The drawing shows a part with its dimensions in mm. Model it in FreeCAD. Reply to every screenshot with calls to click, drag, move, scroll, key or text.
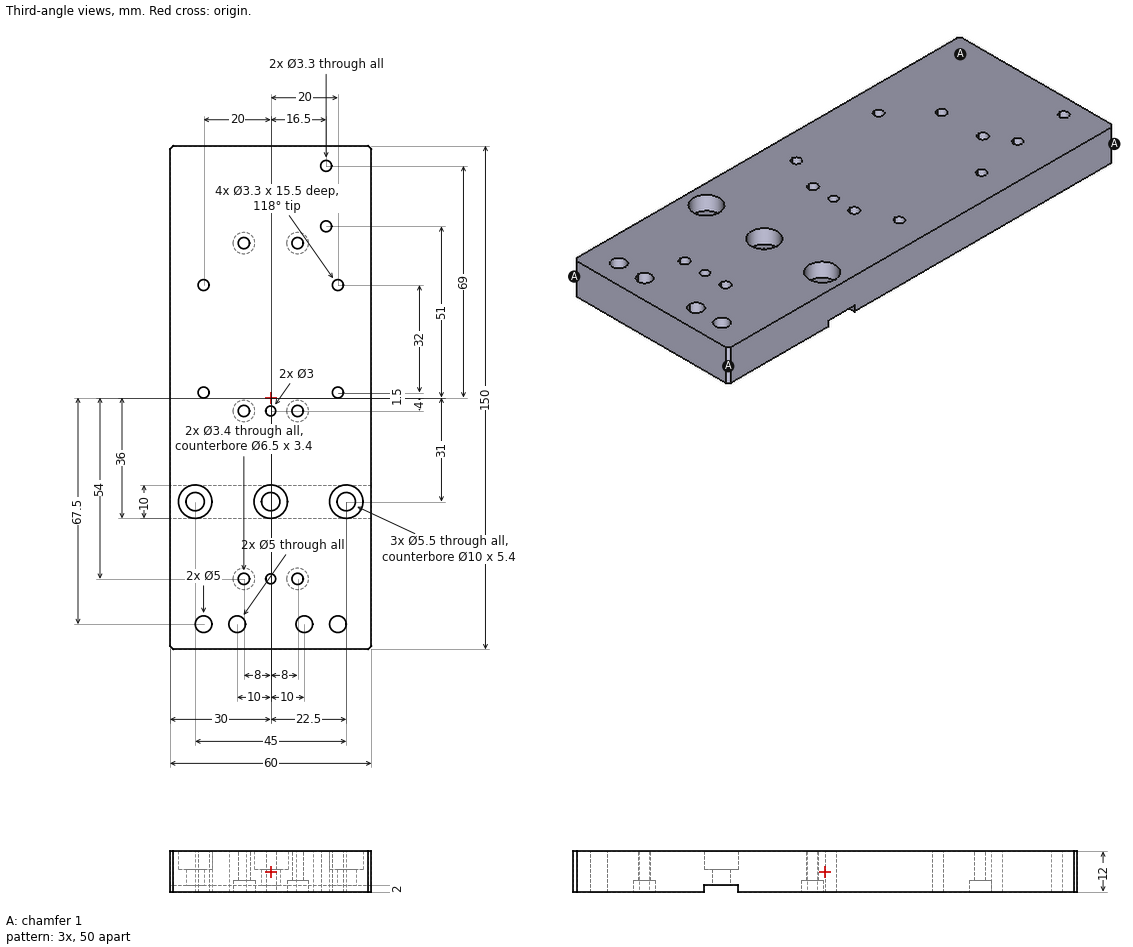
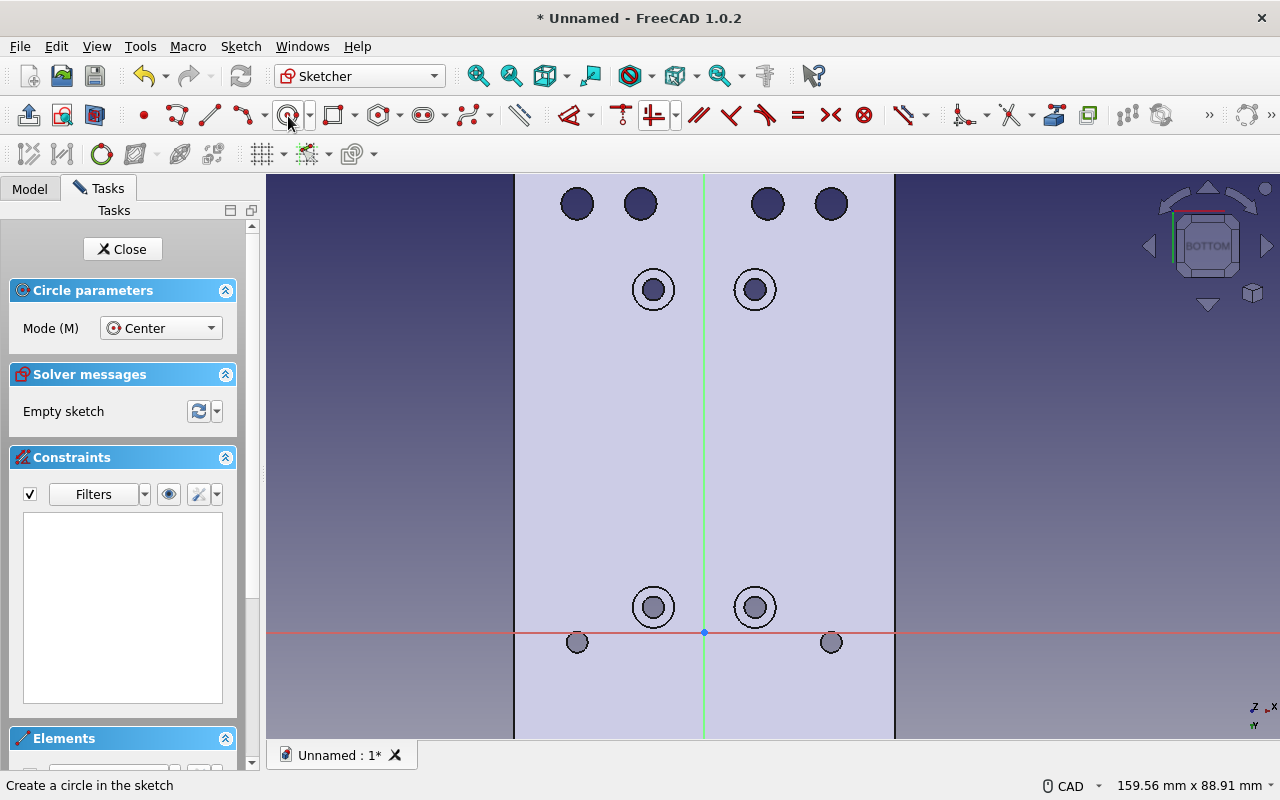
scroll(704, 607, up, 5)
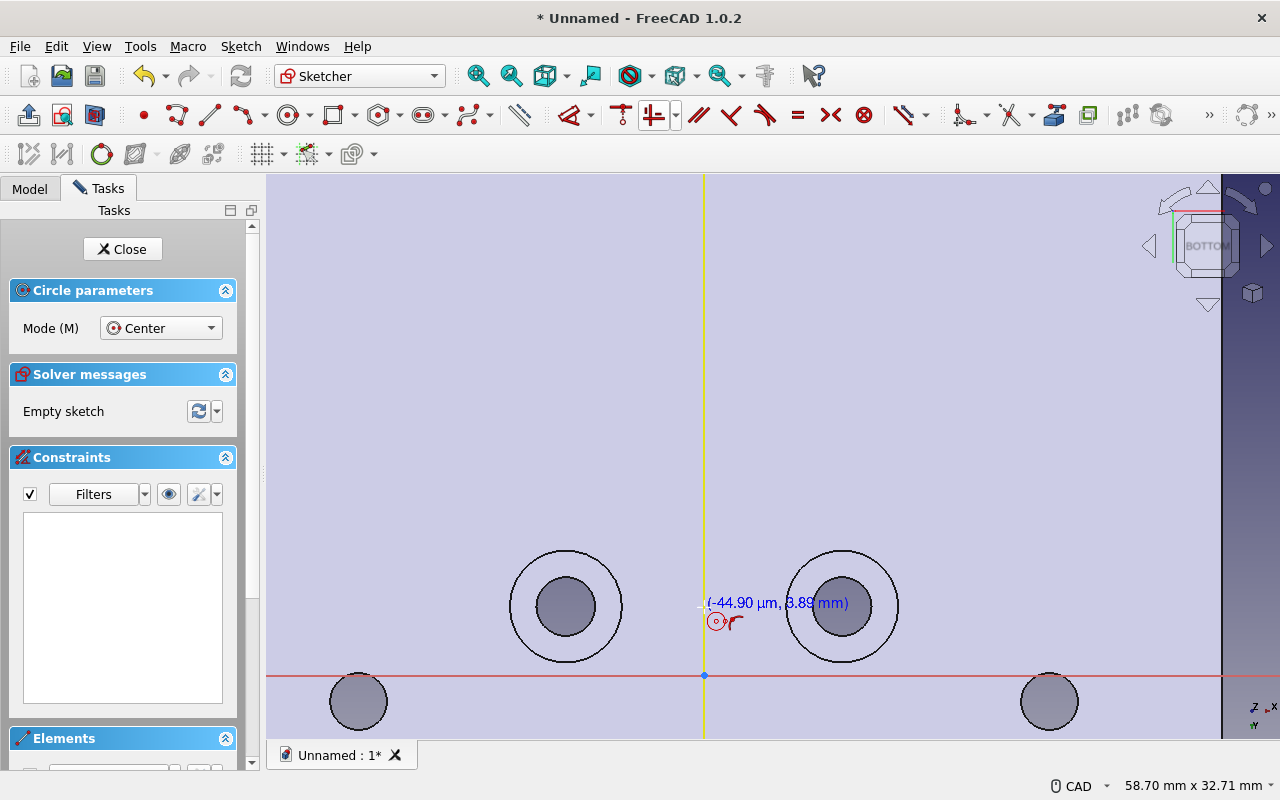
click(704, 607)
click(722, 588)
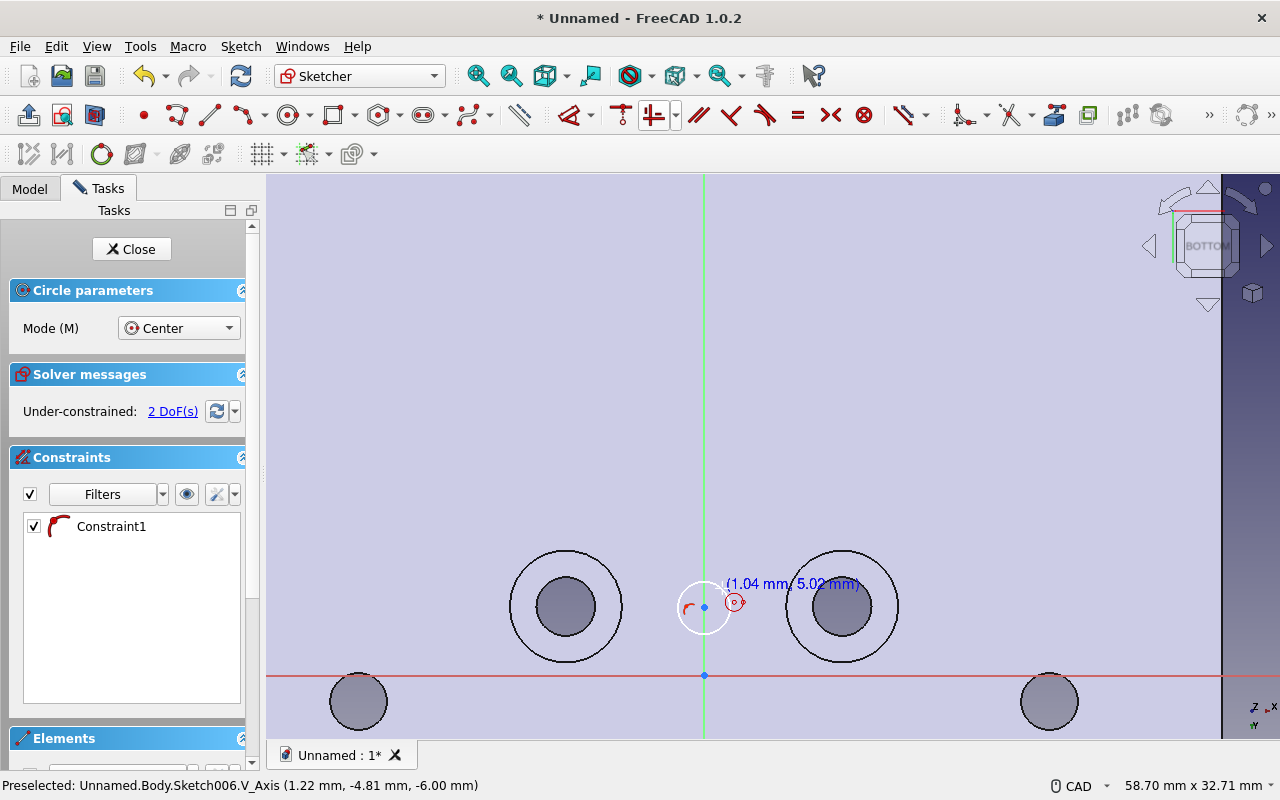
scroll(705, 608, down, 5)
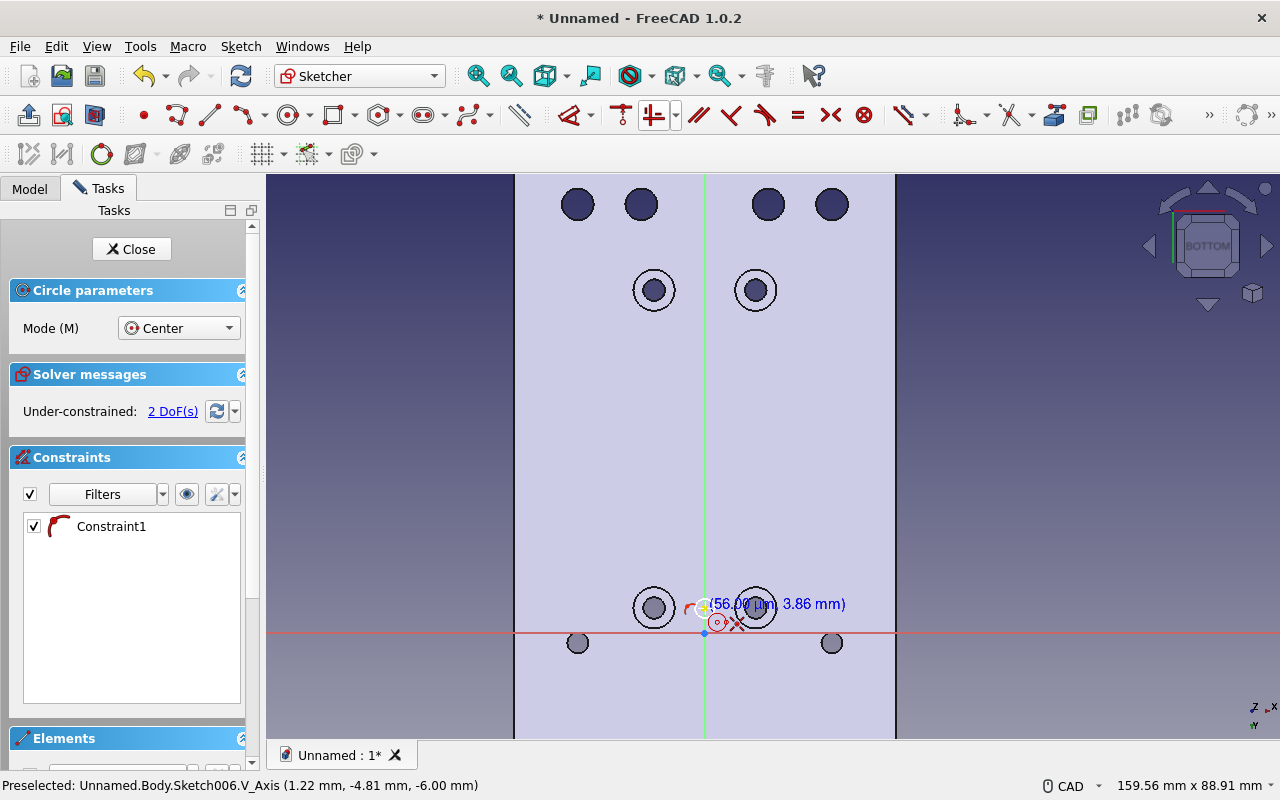
scroll(705, 290, up, 5)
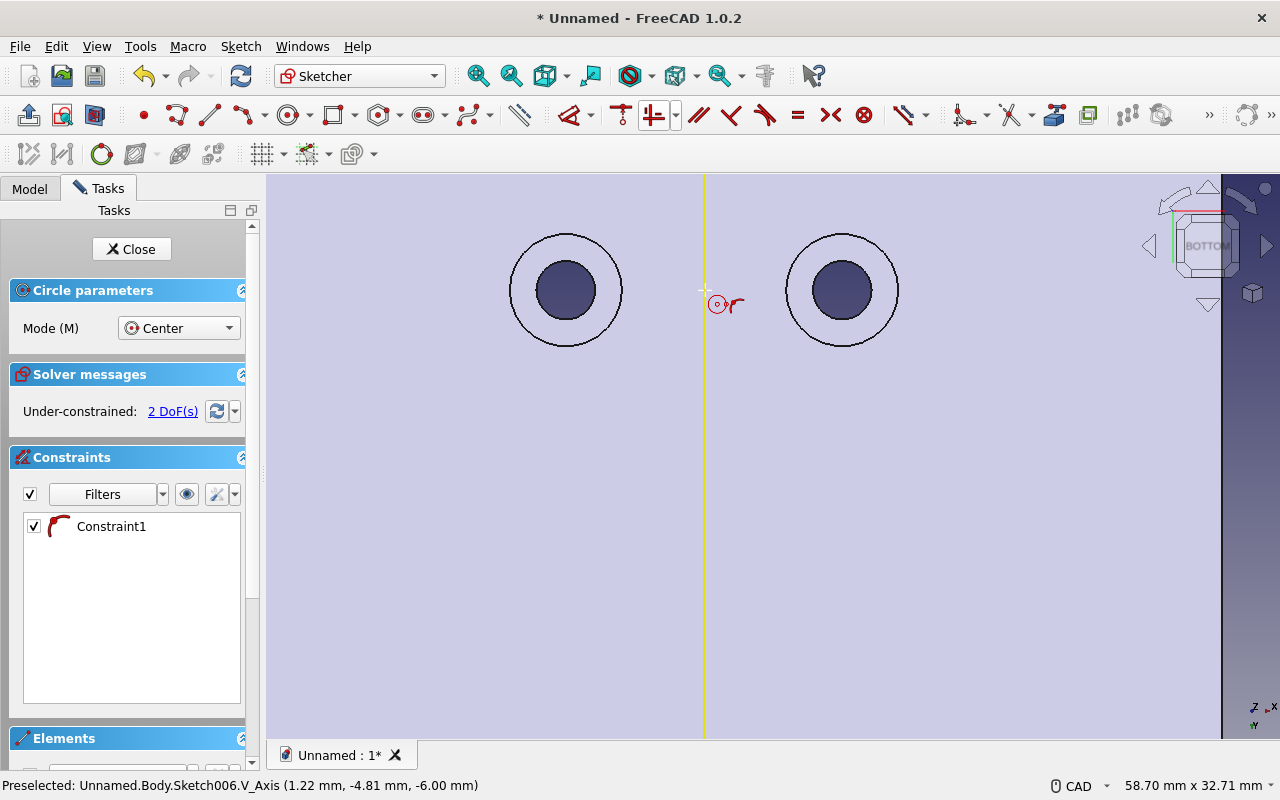
click(704, 290)
click(722, 272)
key(Escape)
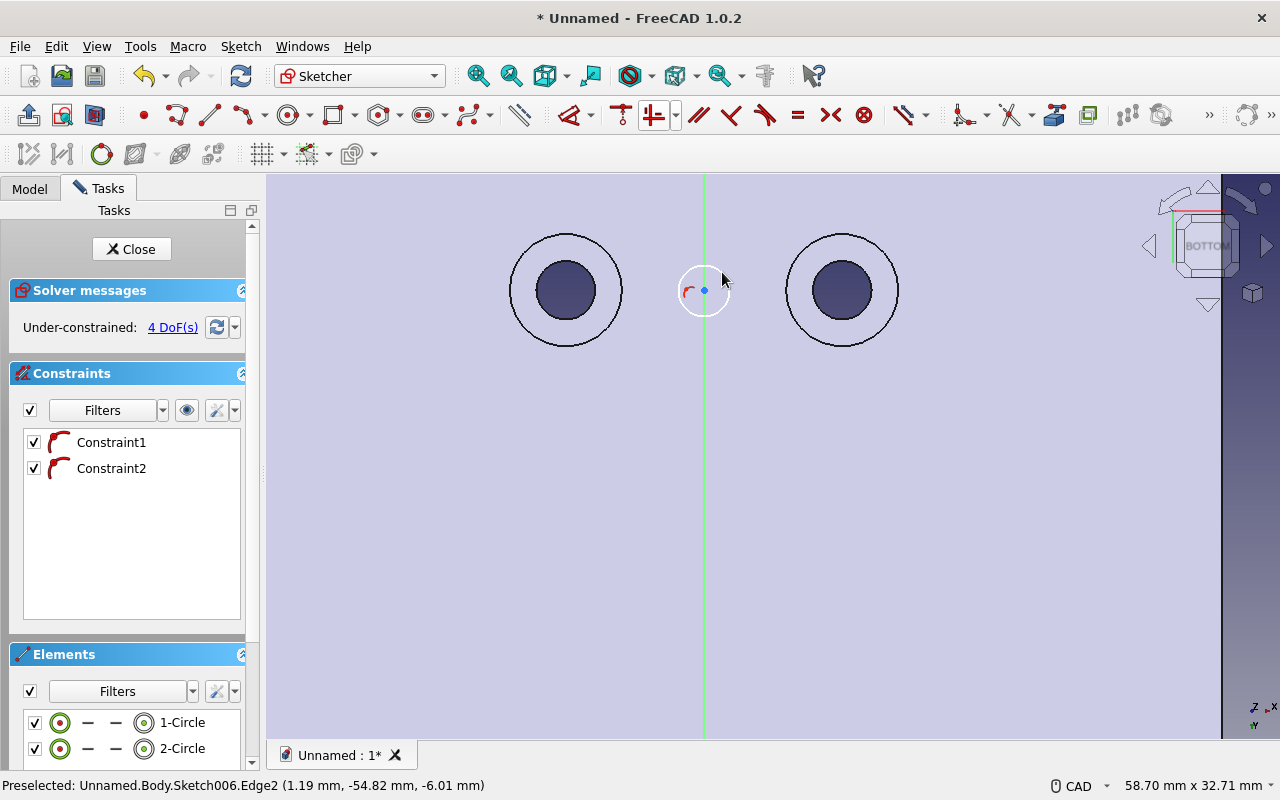
scroll(705, 289, down, 5)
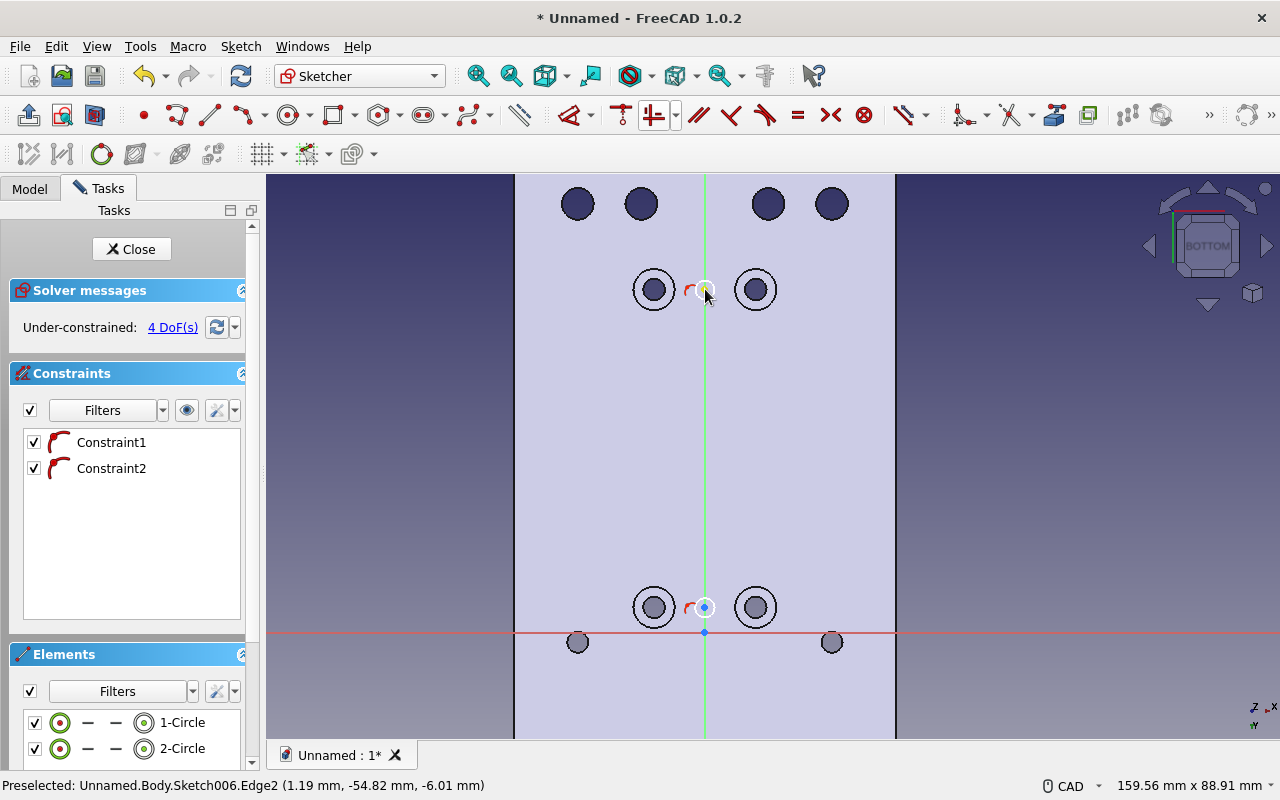
scroll(712, 601, up, 4)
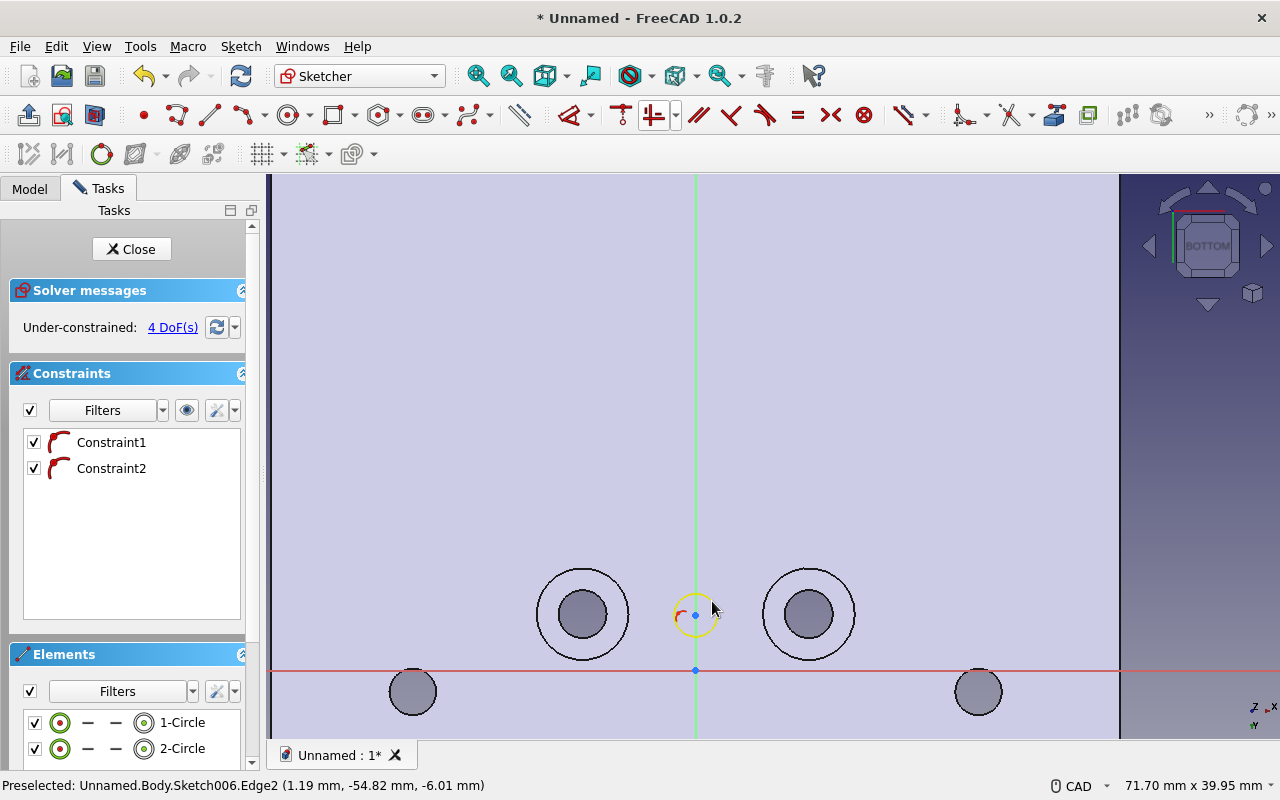
click(711, 600)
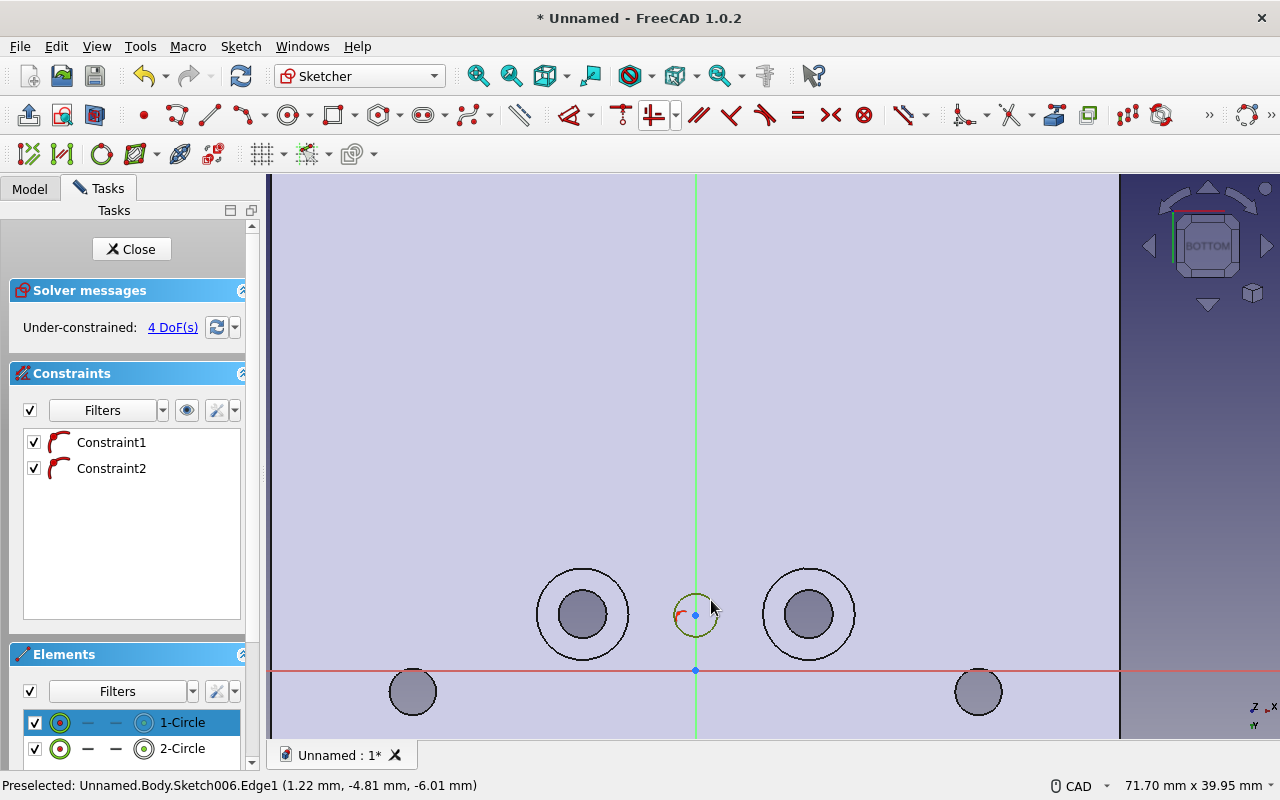
scroll(712, 602, down, 4)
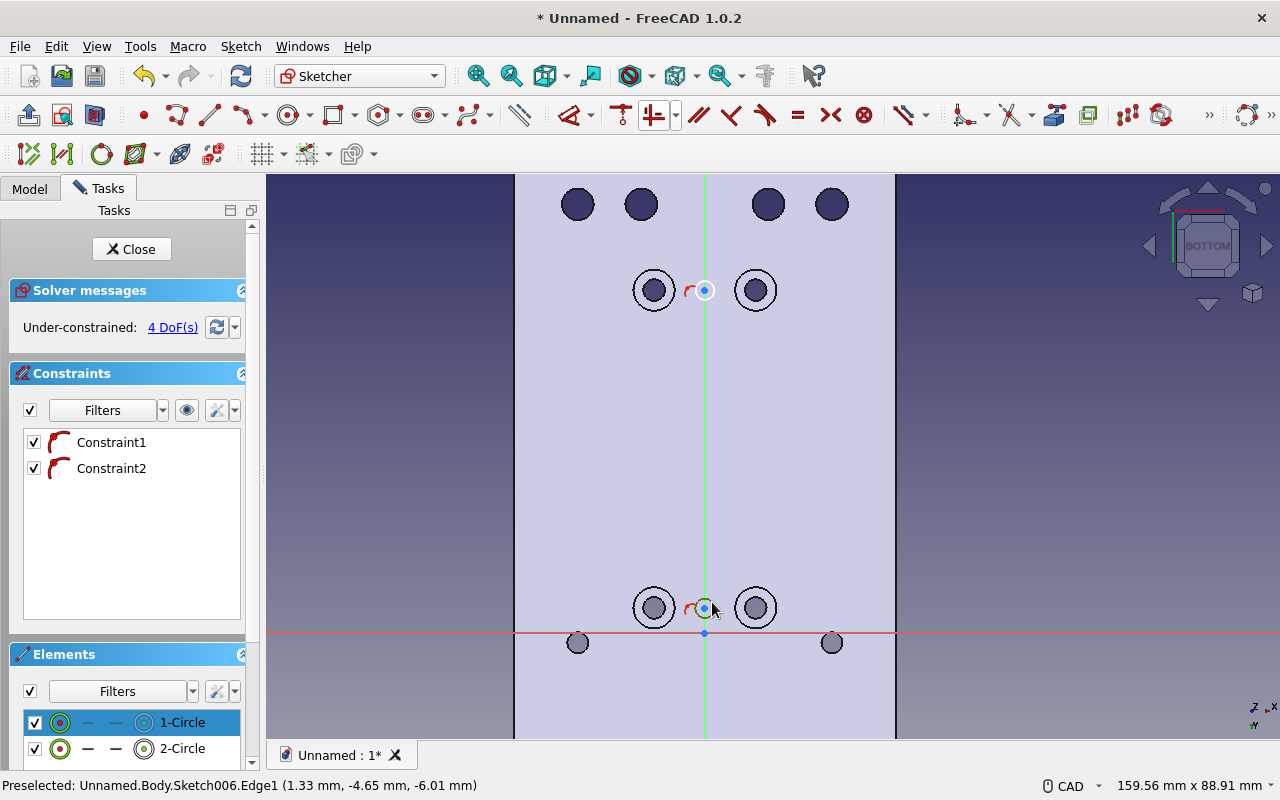
scroll(712, 284, up, 4)